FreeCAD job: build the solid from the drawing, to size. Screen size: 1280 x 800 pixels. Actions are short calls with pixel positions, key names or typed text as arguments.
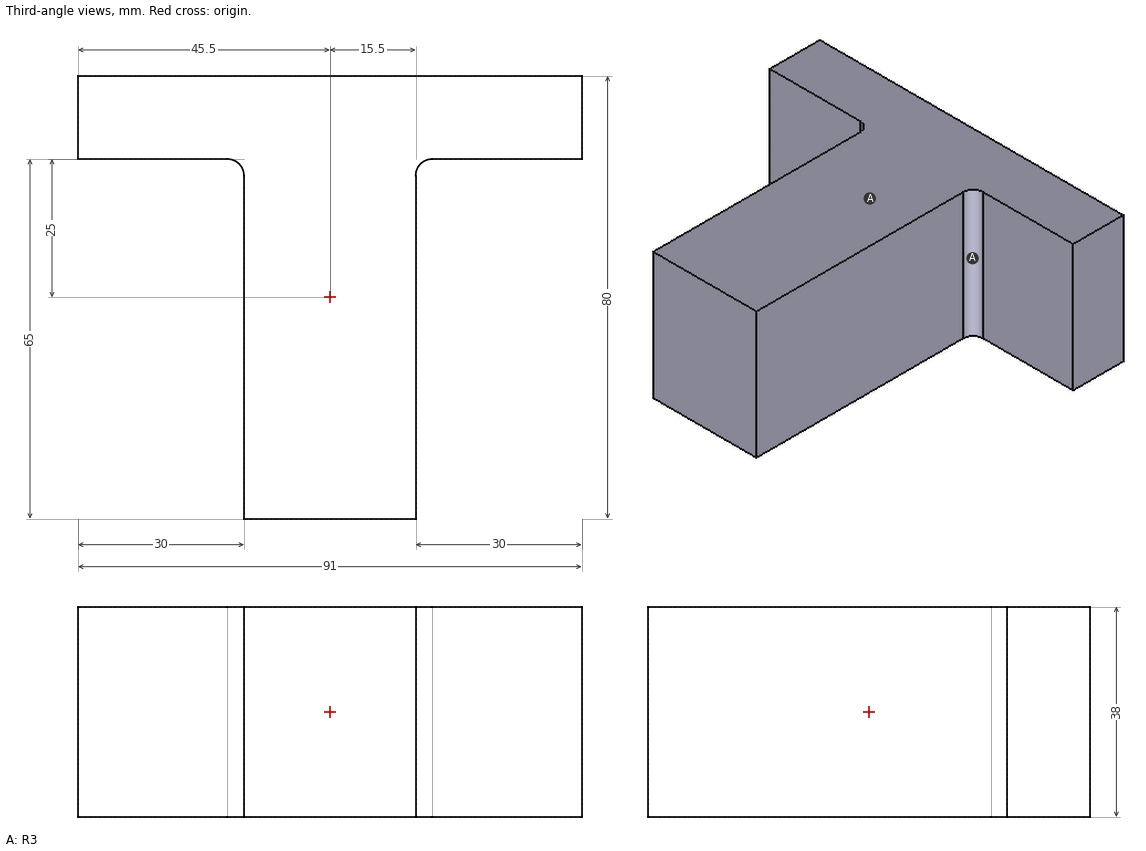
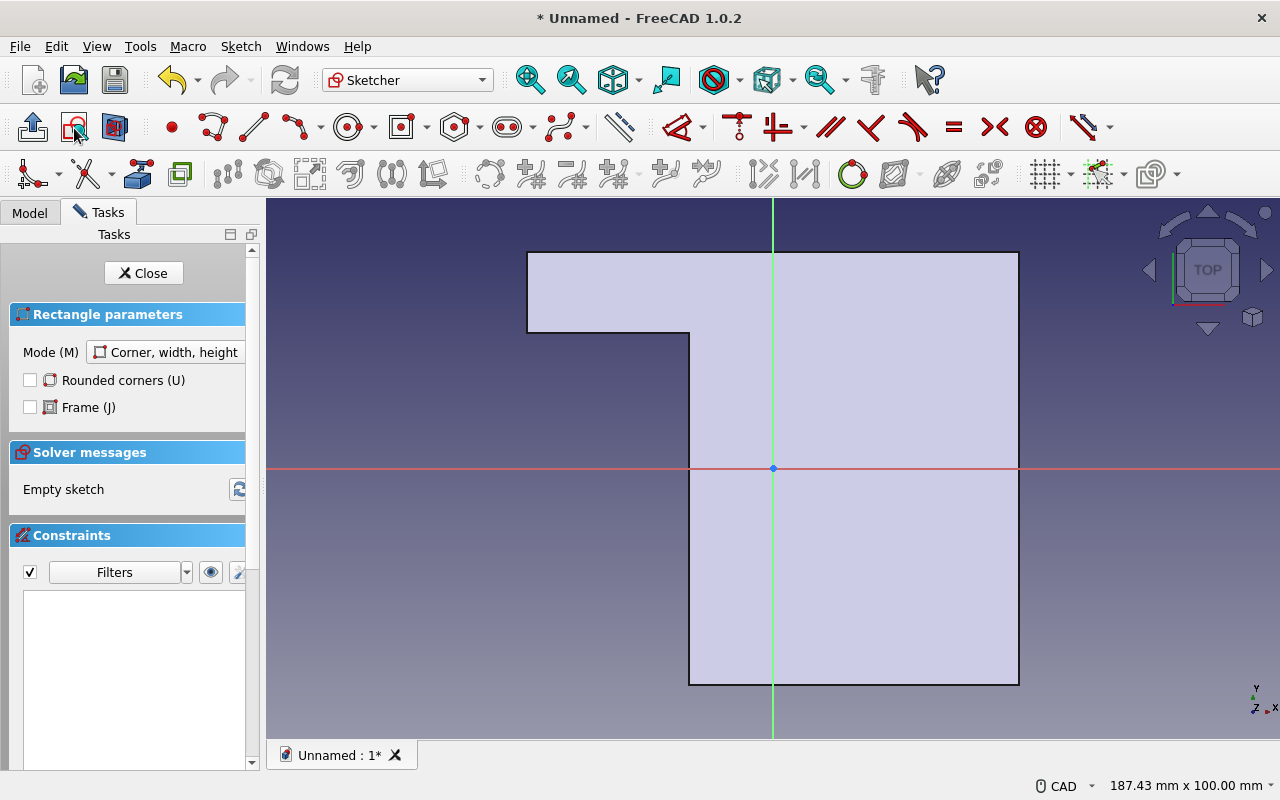
click(857, 333)
move(1019, 685)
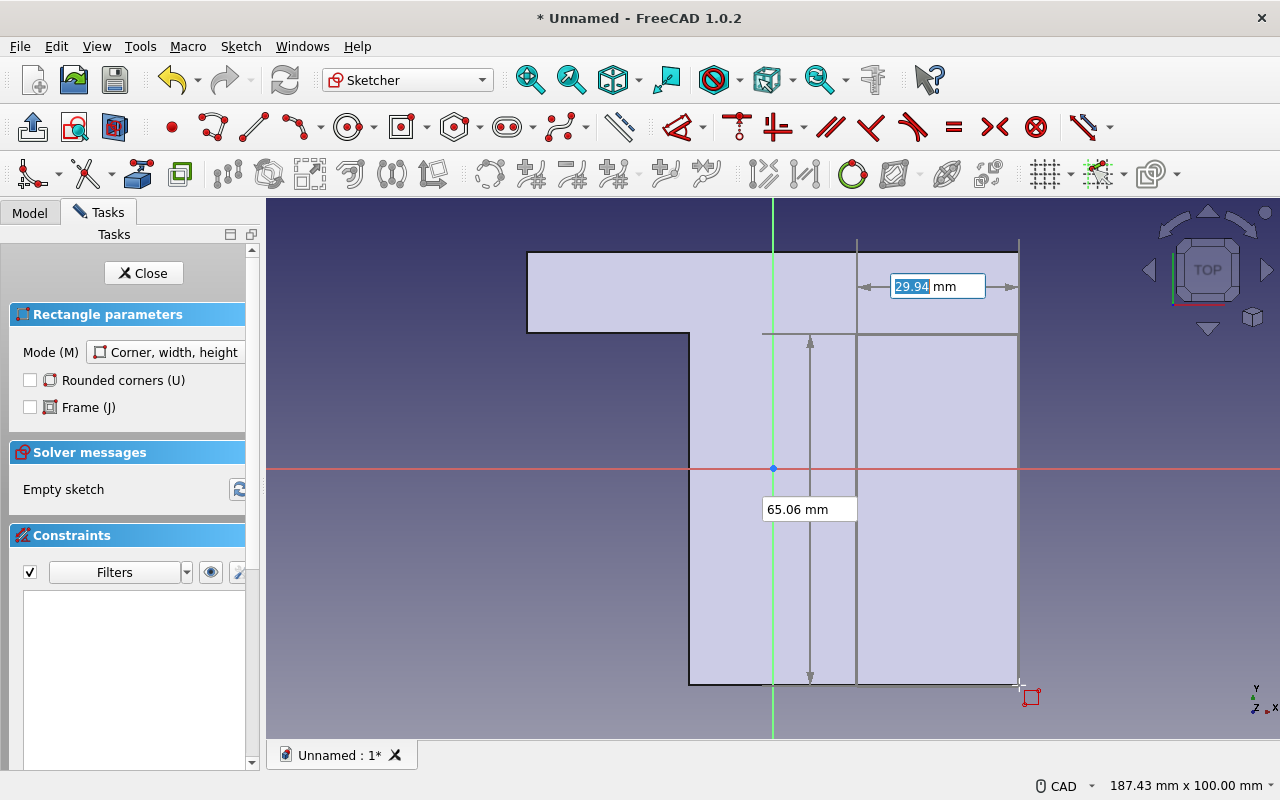
text(30)
key(Tab)
text(65)
key(Return)
key(Escape)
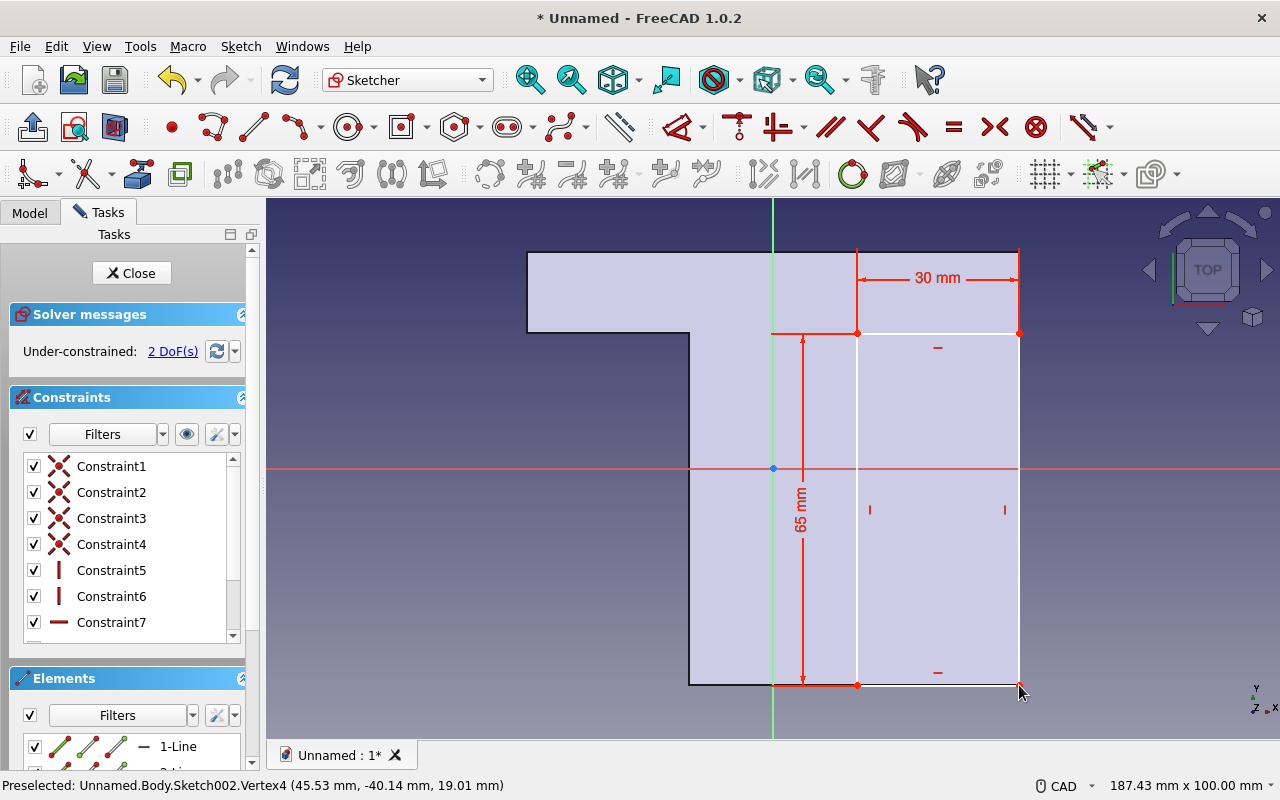
click(676, 128)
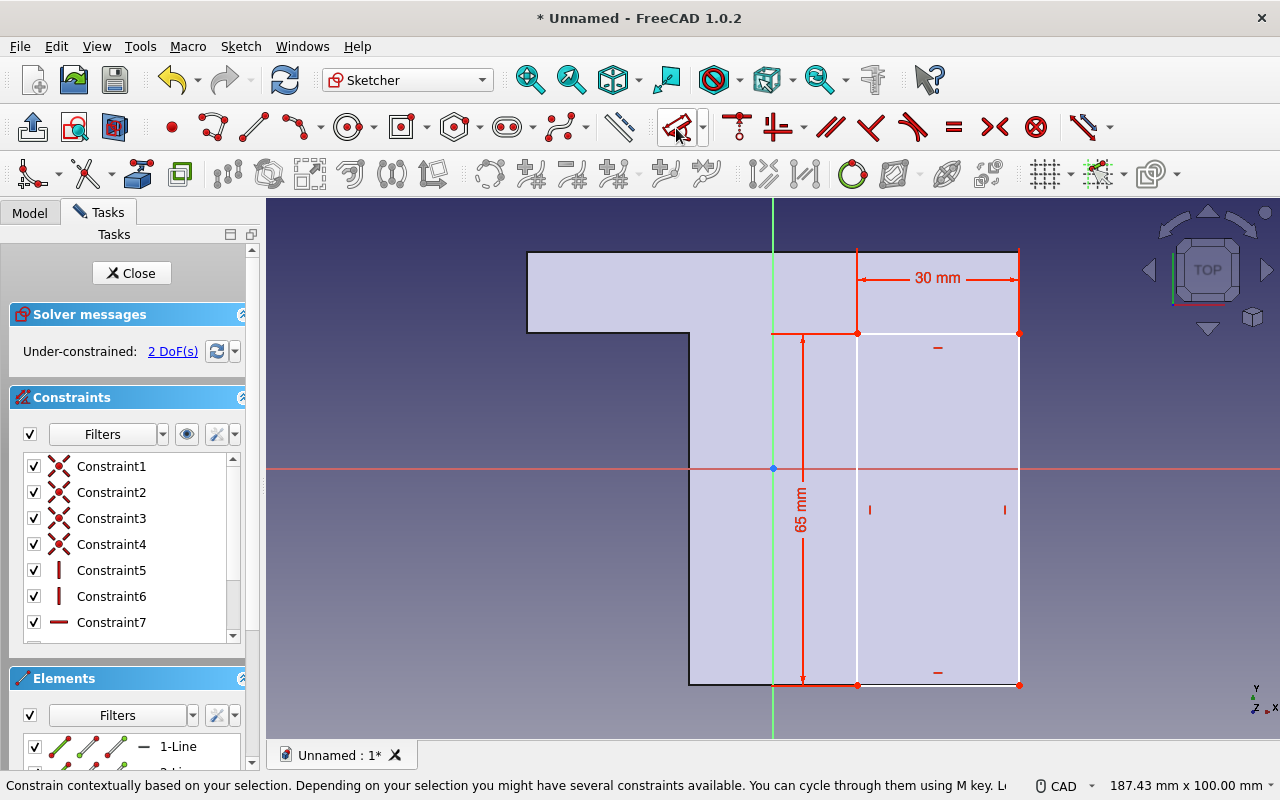
click(857, 334)
click(739, 401)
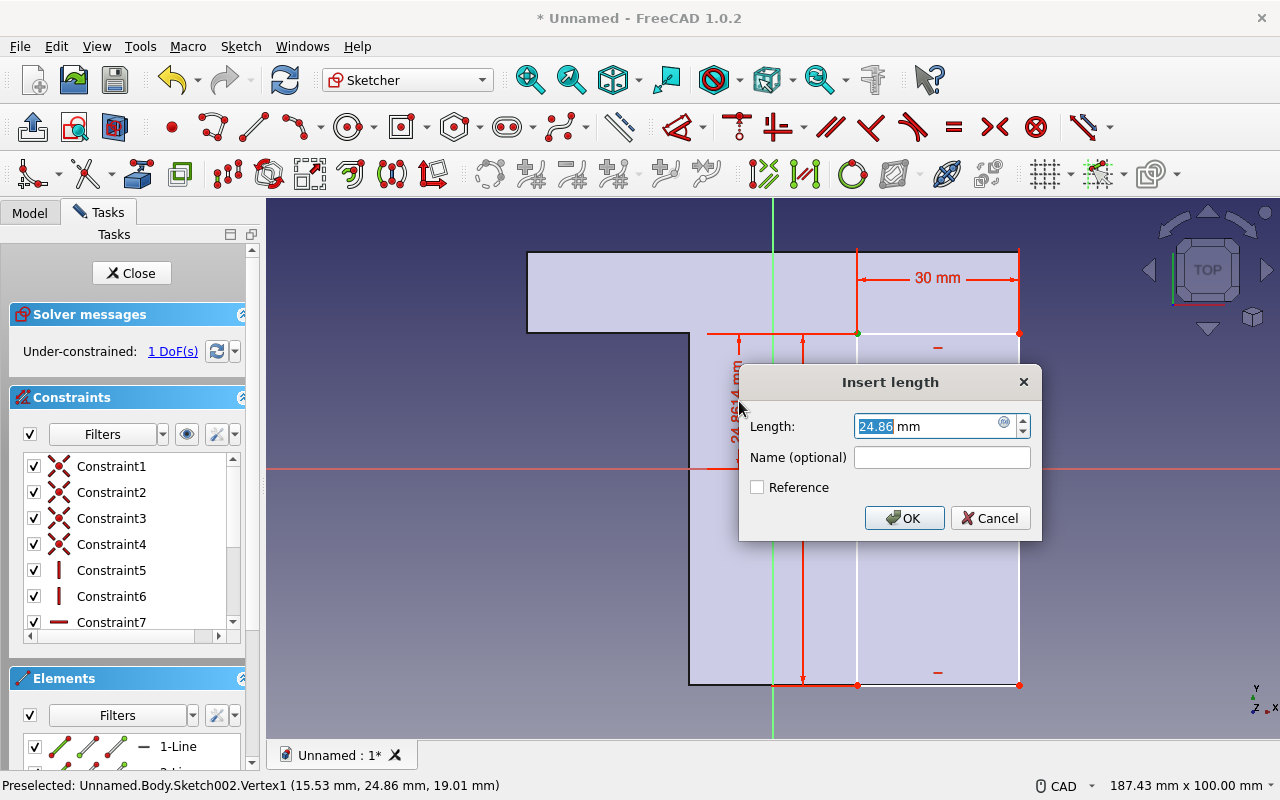
text(25)
key(Return)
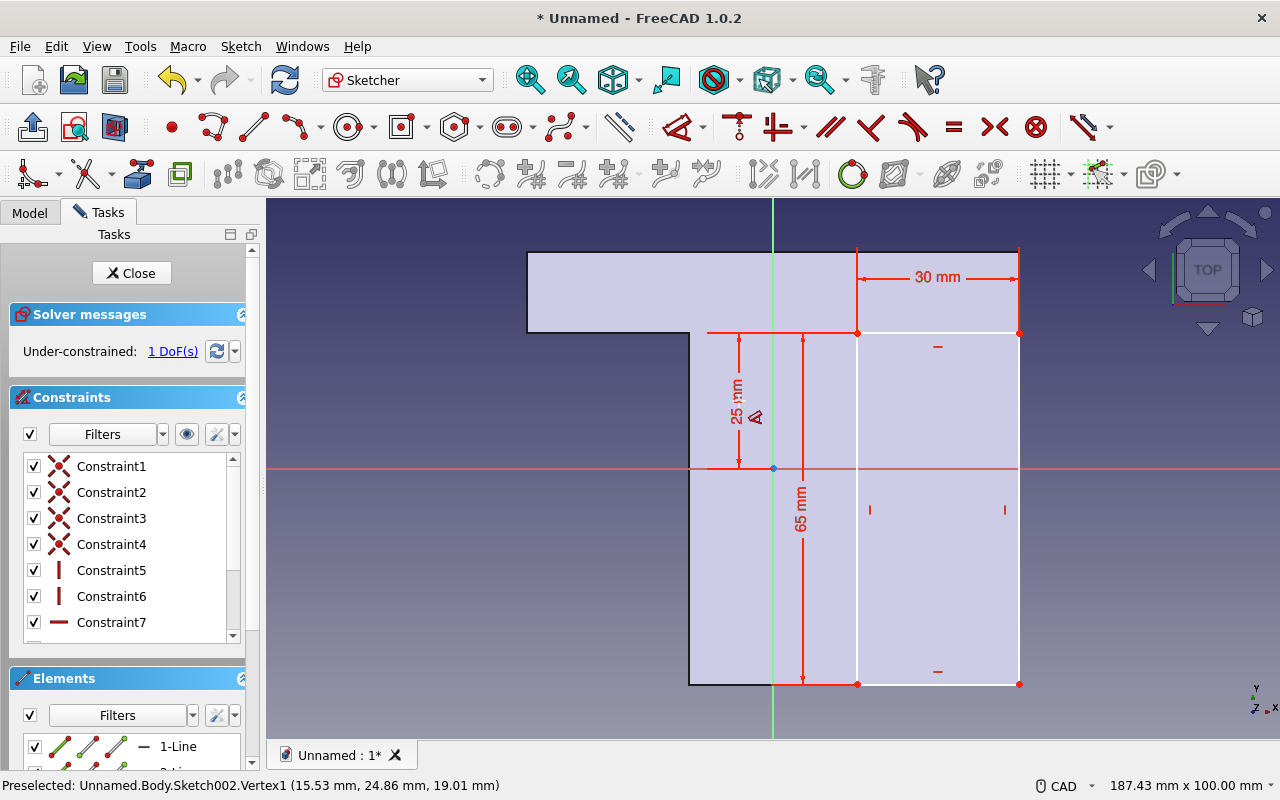
click(857, 333)
click(815, 299)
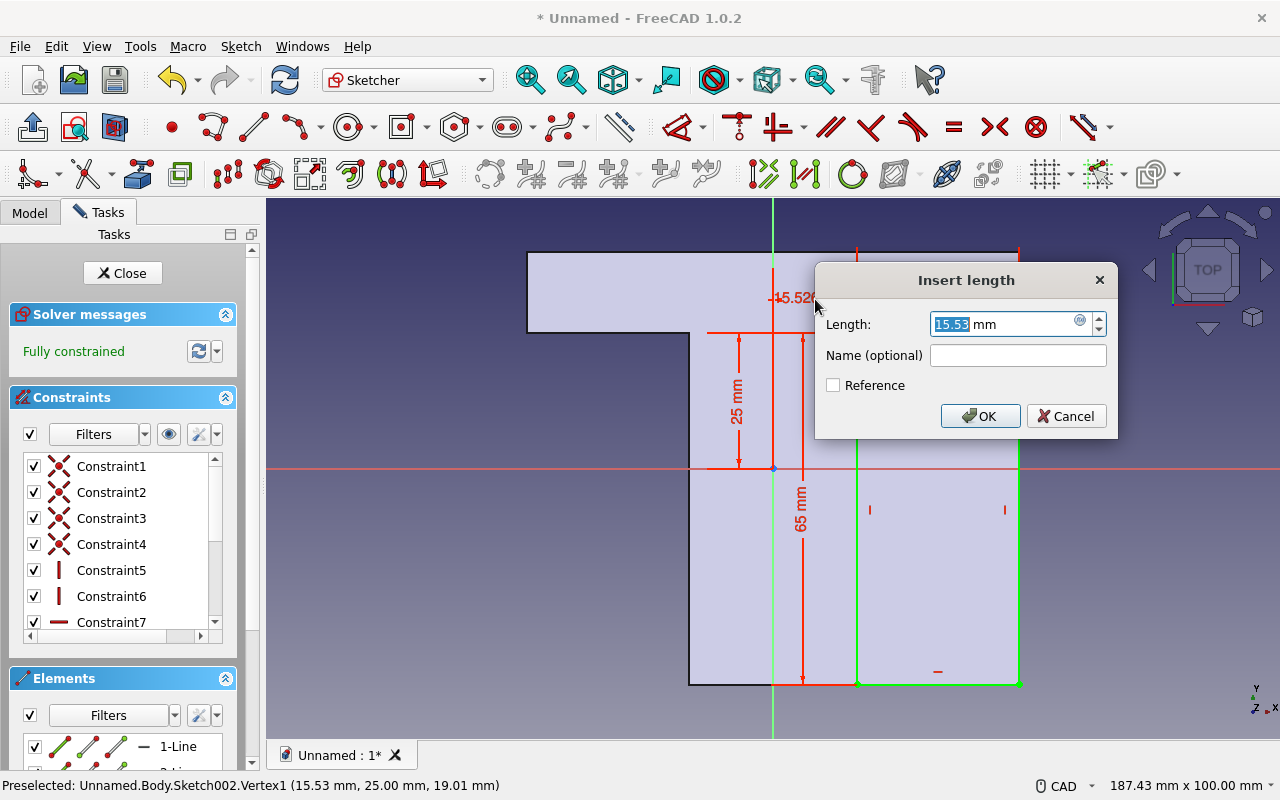
text(15.5)
key(Return)
key(Escape)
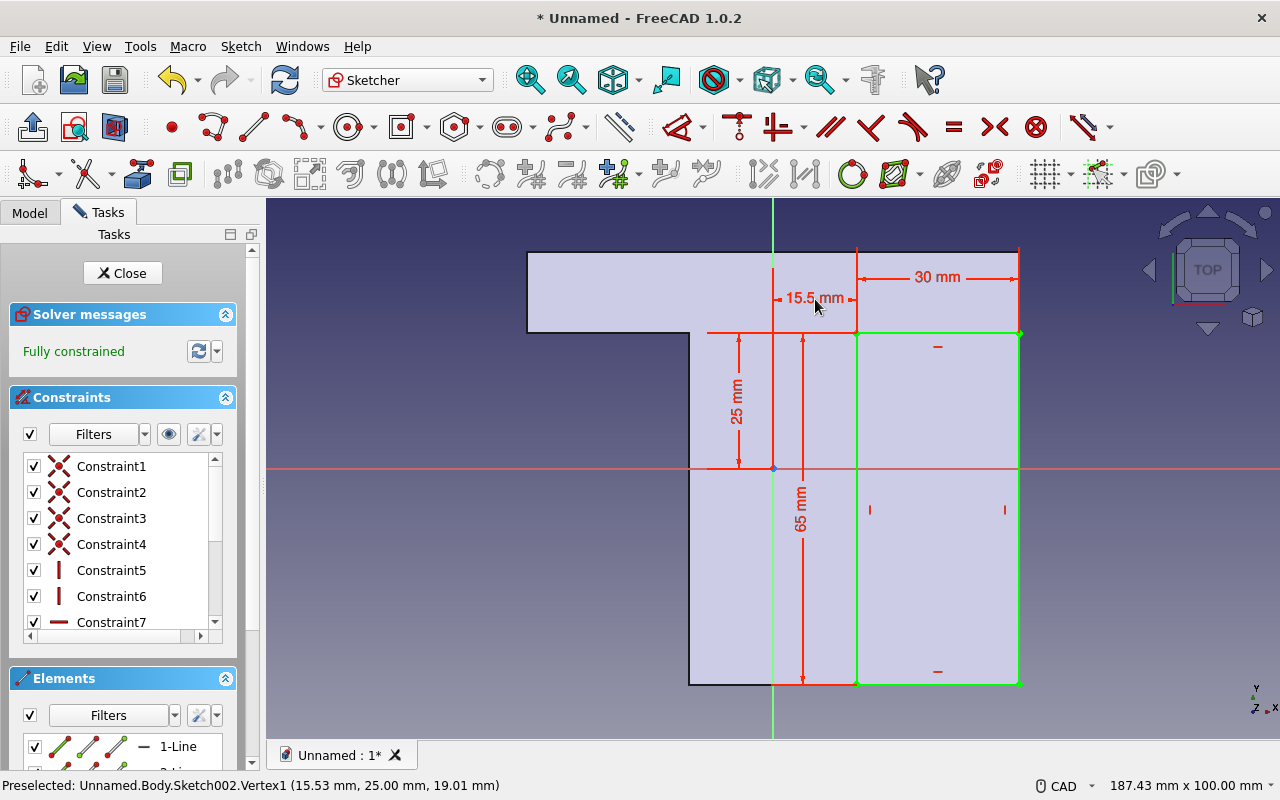
click(123, 273)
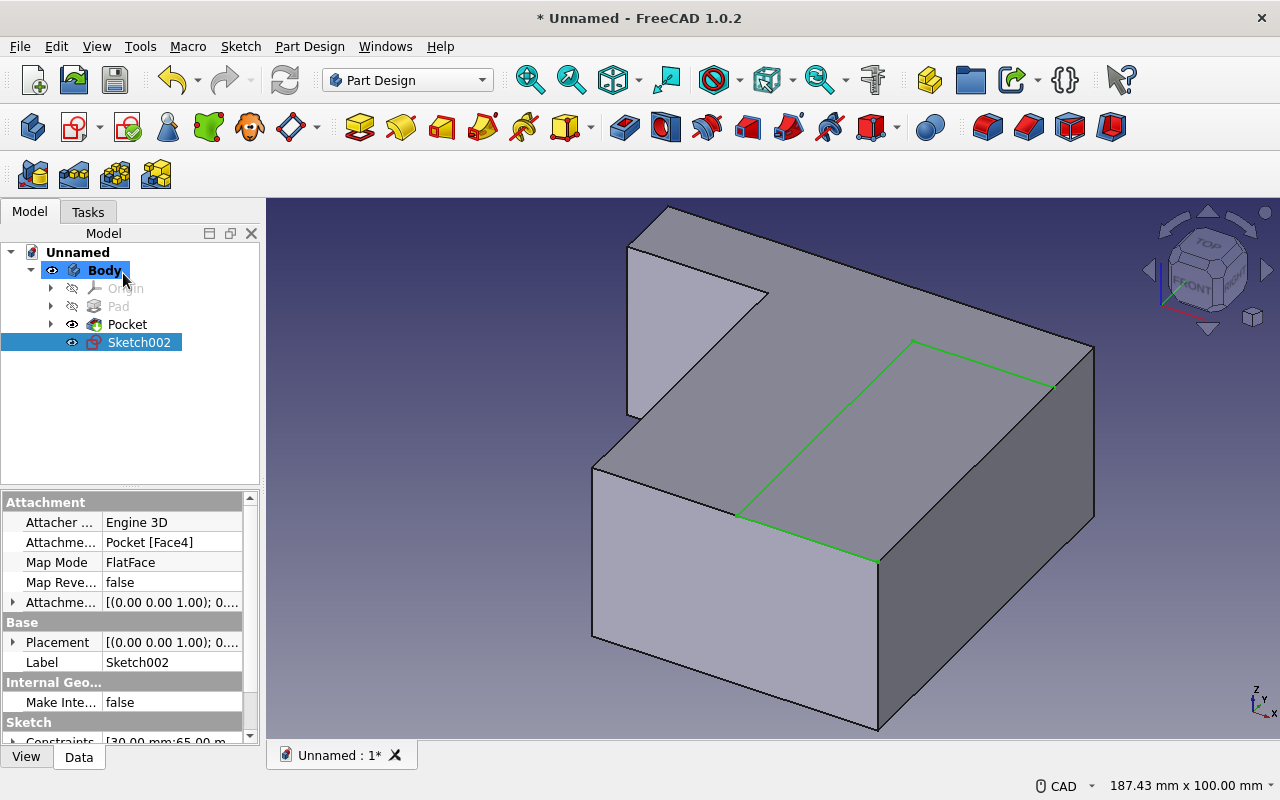
click(625, 128)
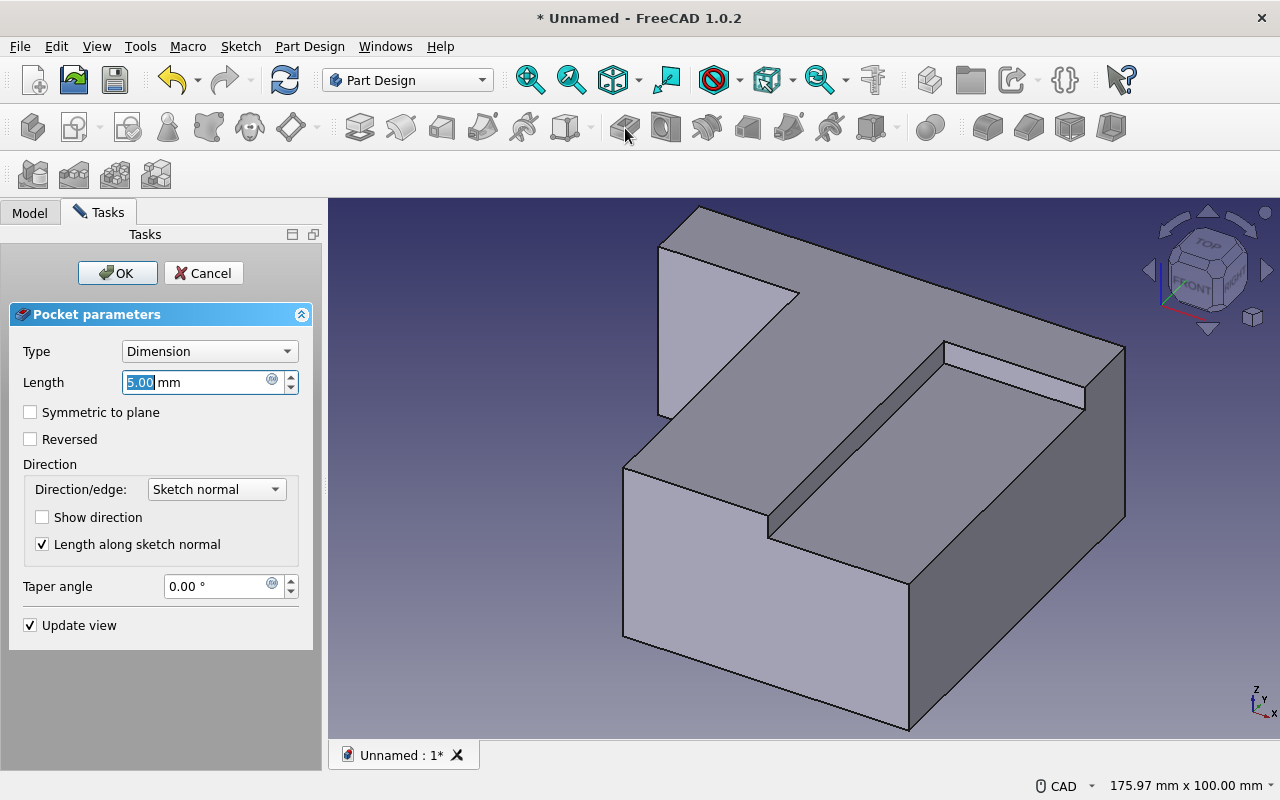
click(210, 352)